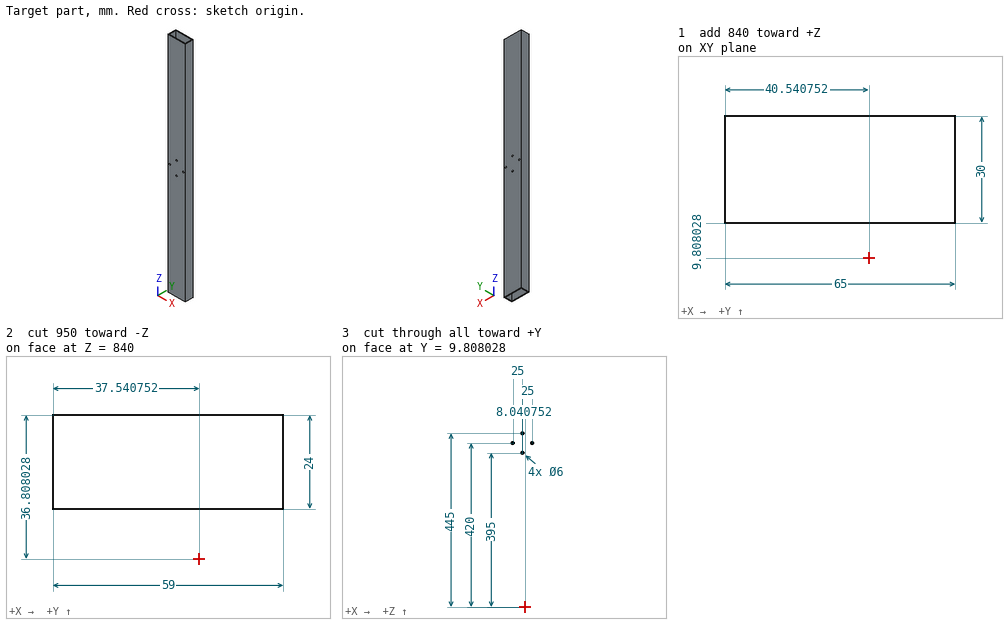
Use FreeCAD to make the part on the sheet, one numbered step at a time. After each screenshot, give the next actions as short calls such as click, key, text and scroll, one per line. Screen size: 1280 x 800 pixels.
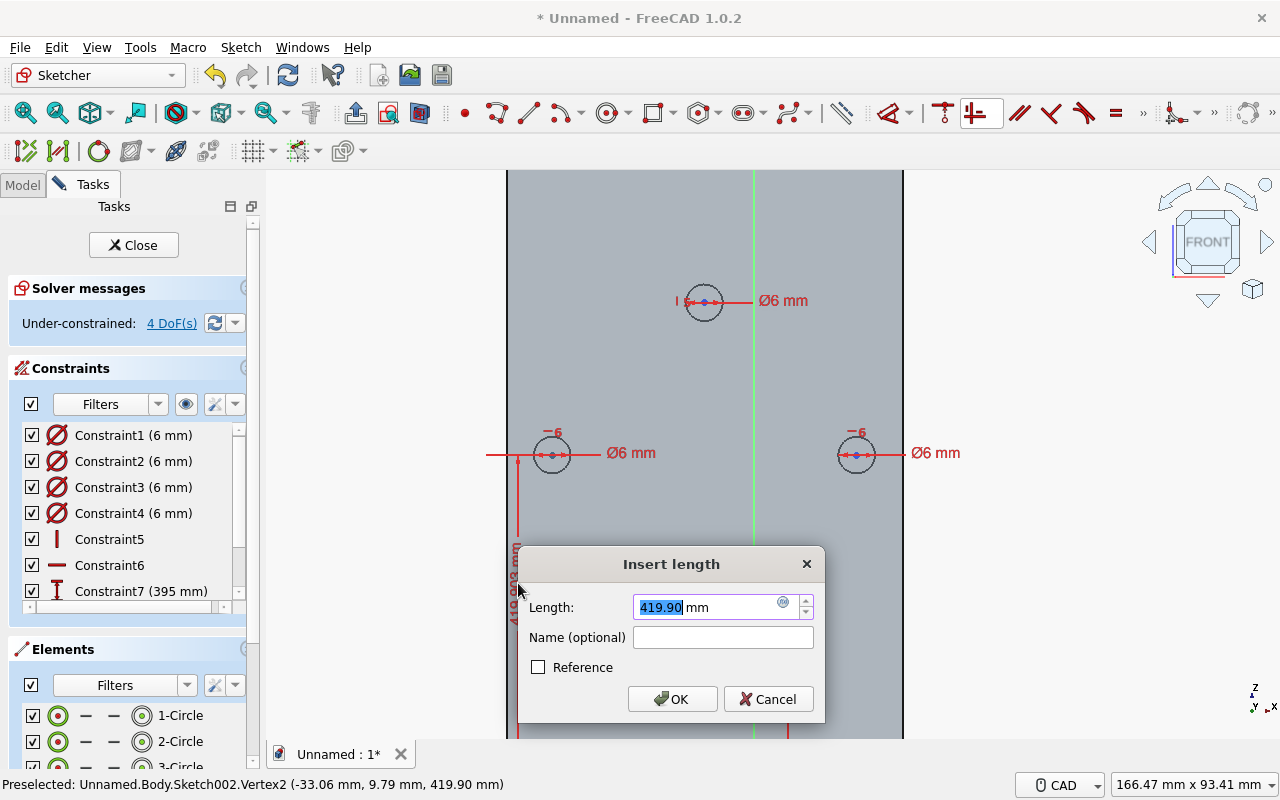
text(420)
key(Return)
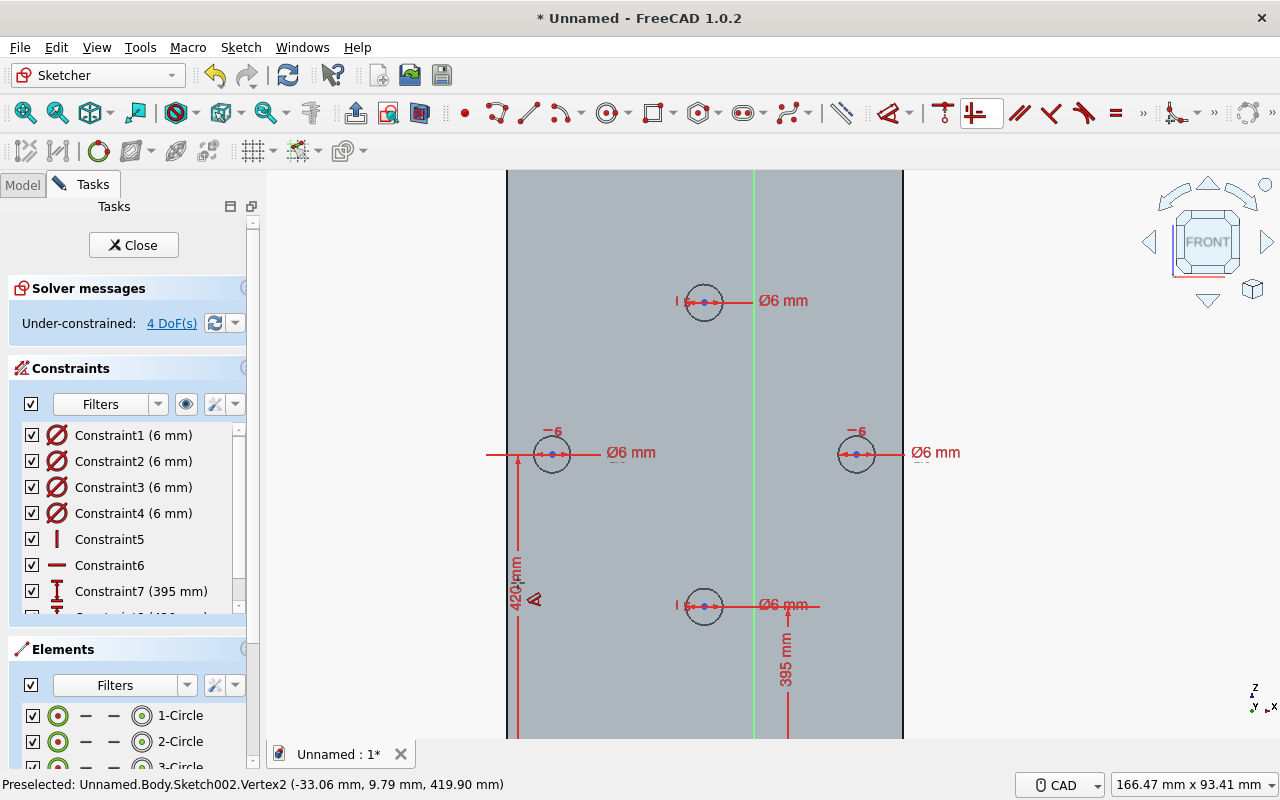
click(704, 303)
click(788, 507)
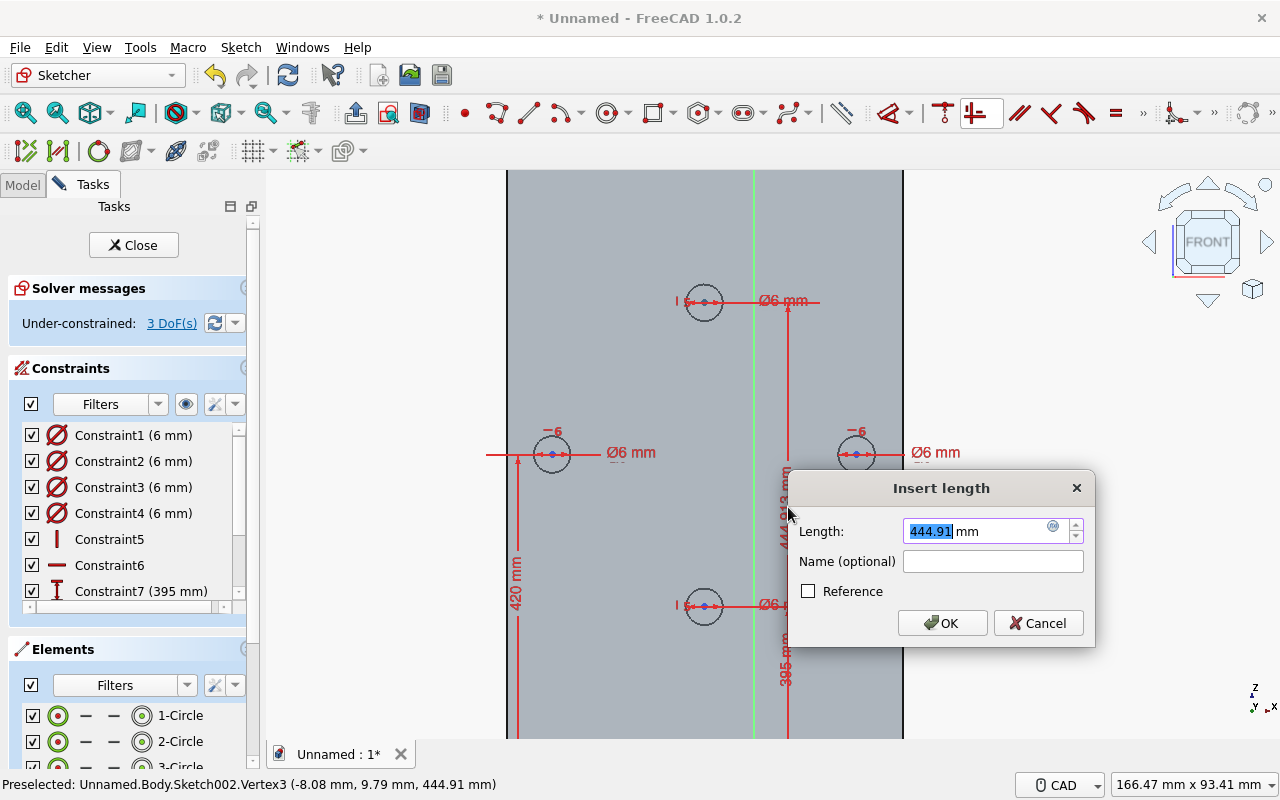
text(445)
key(Return)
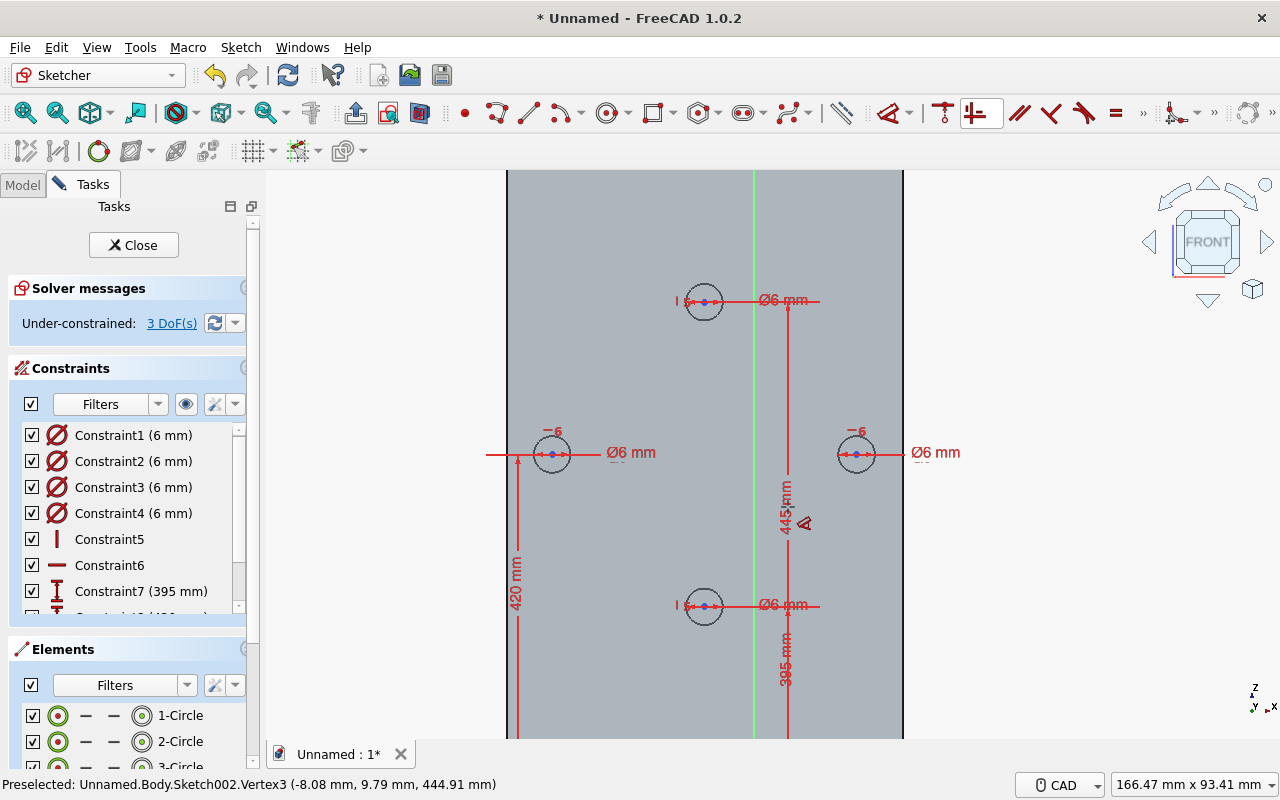
click(704, 607)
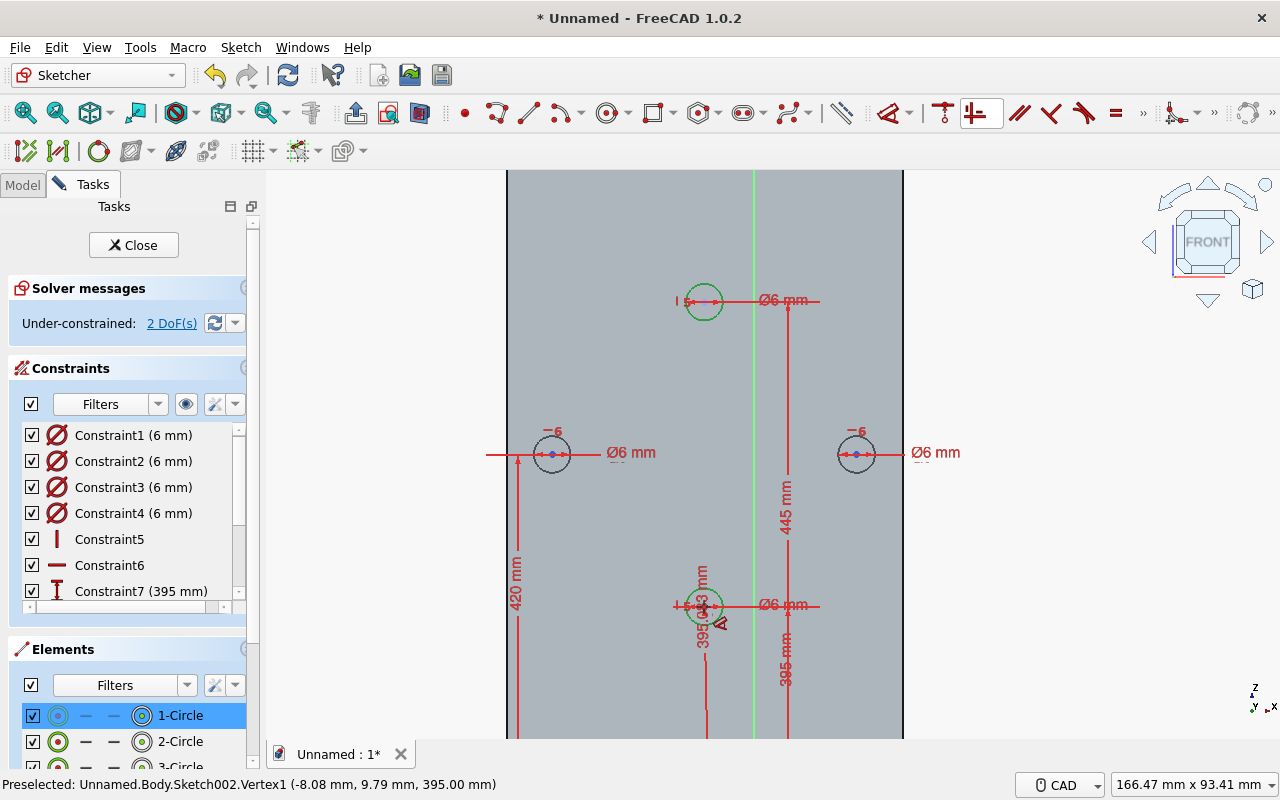
click(552, 454)
click(628, 641)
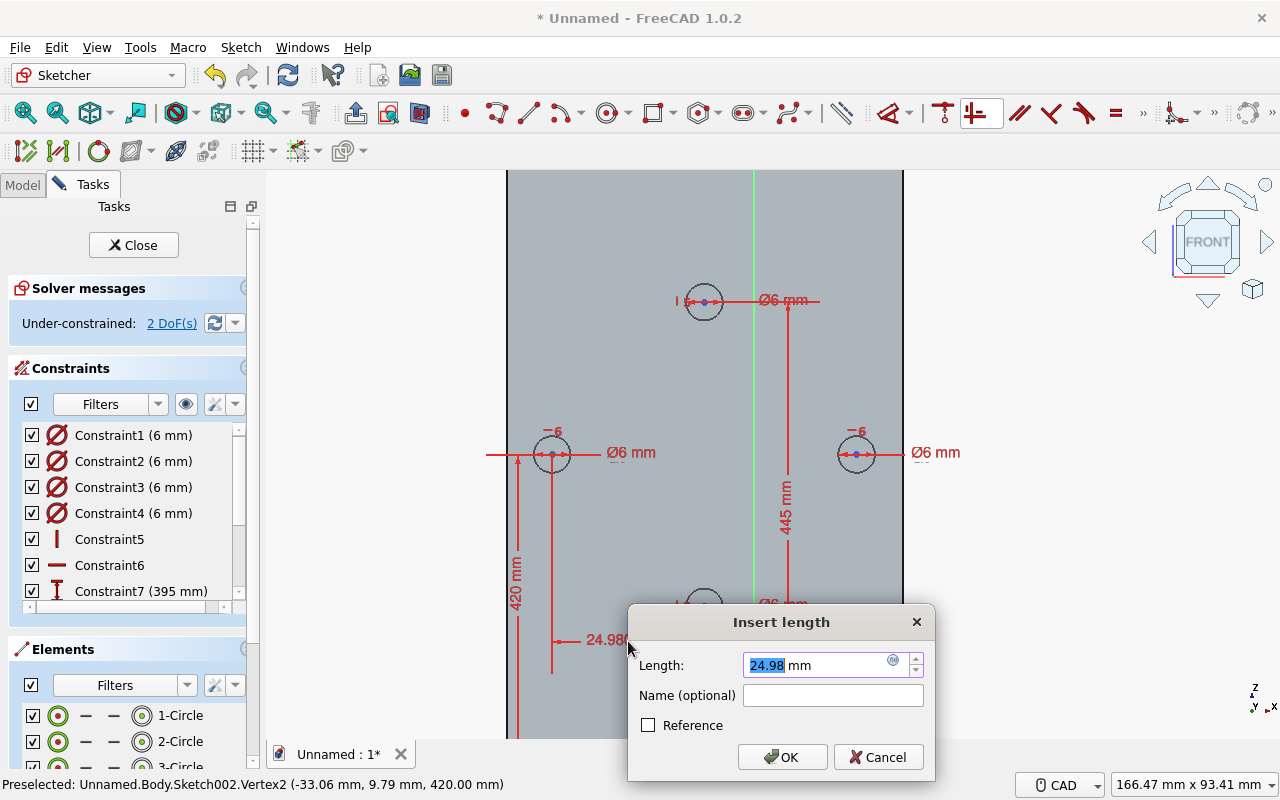
text(25)
key(Return)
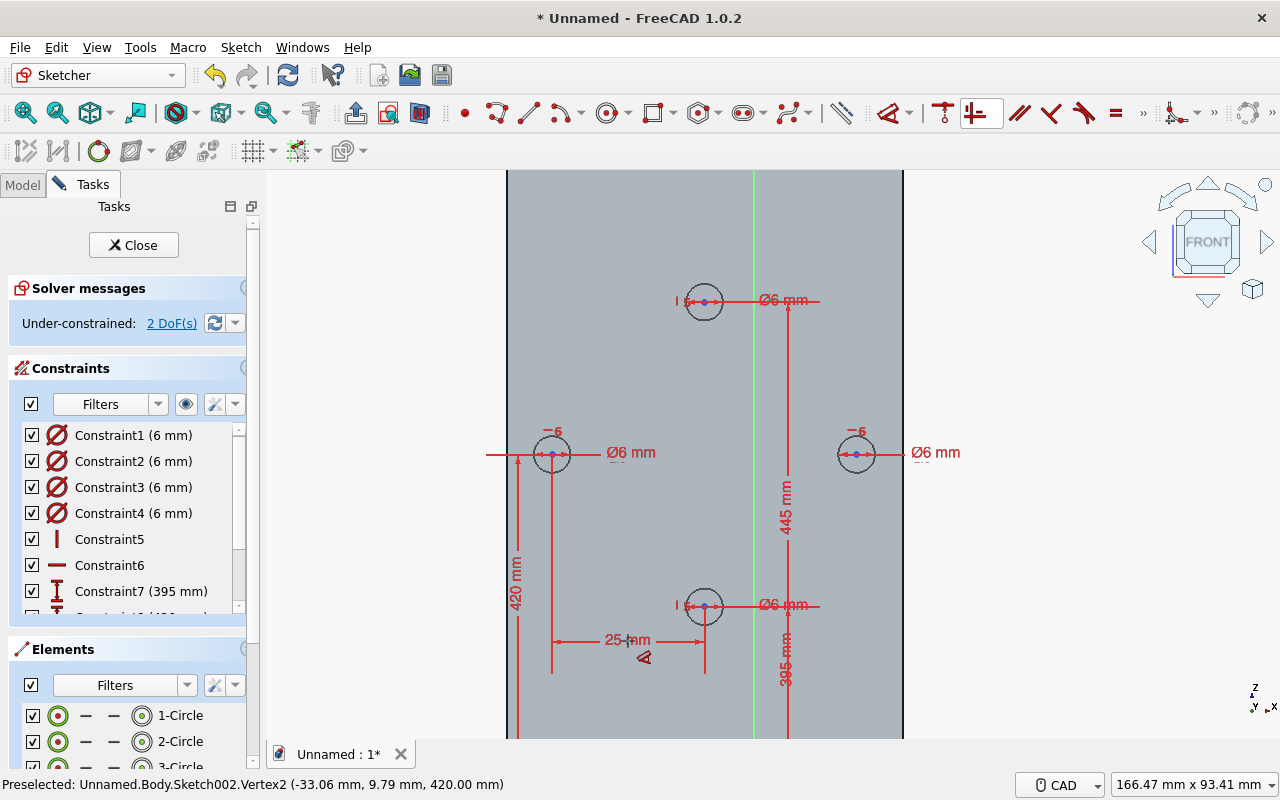
click(705, 607)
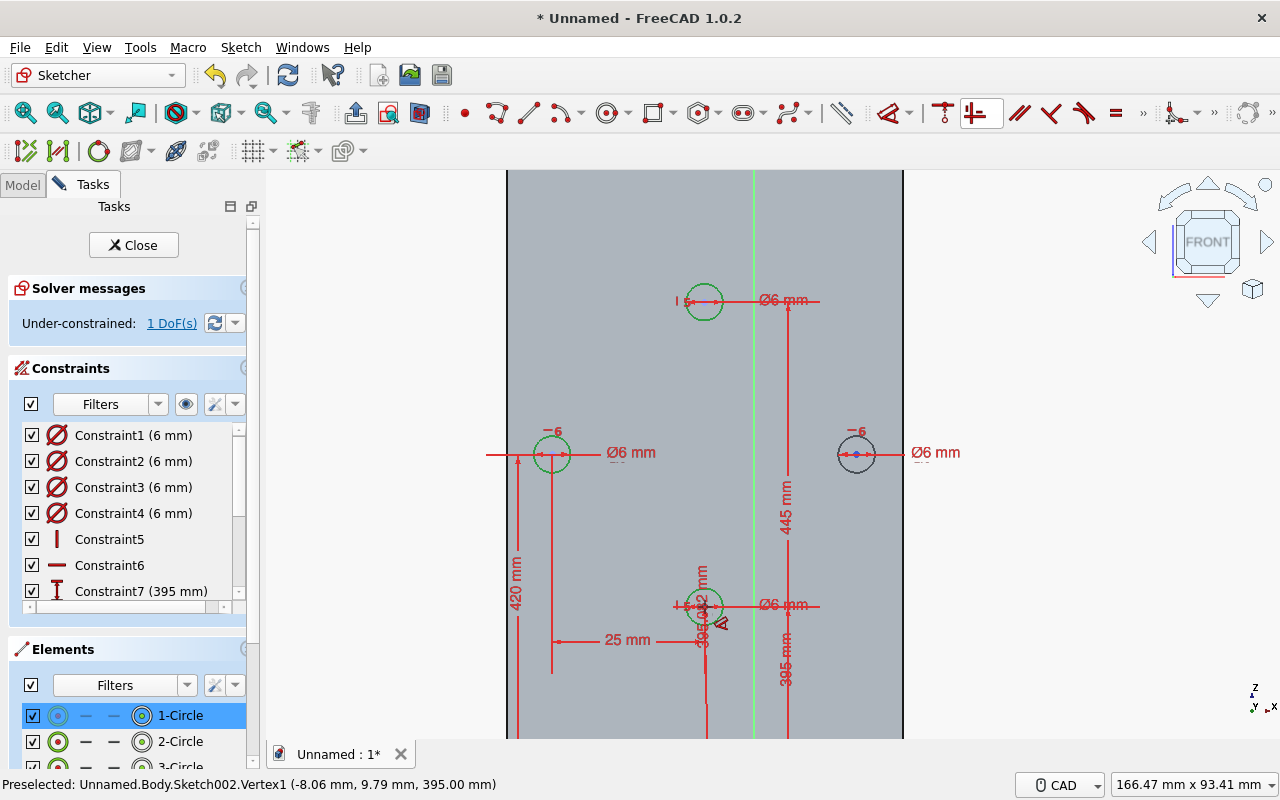
click(857, 454)
click(781, 420)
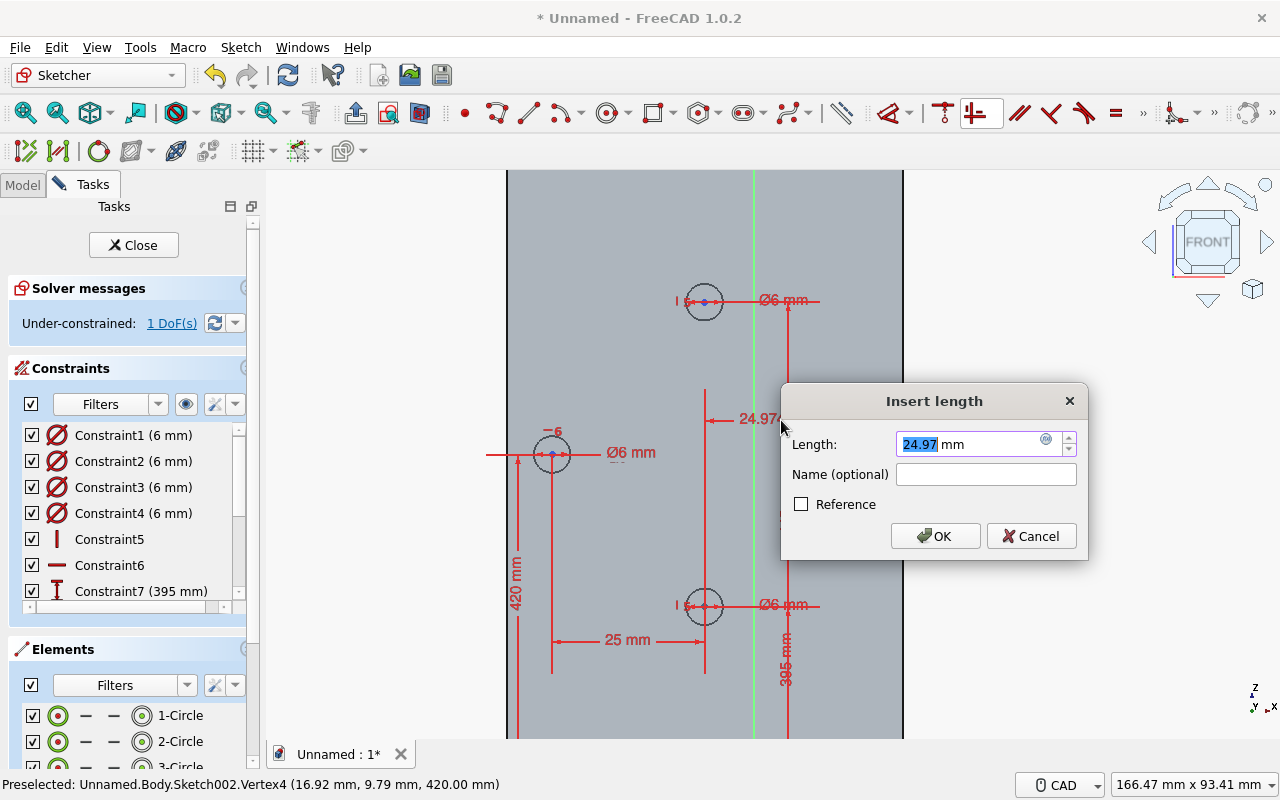
text(25)
key(Return)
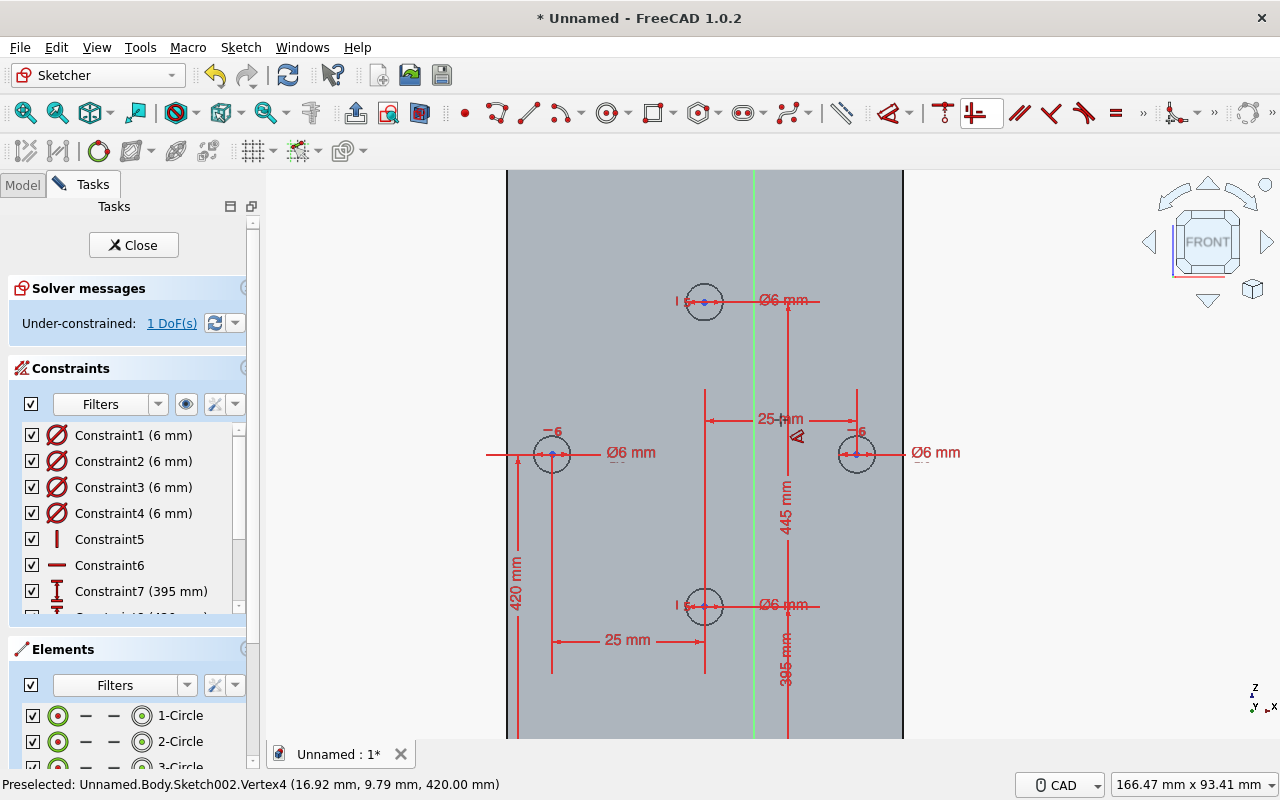
click(705, 607)
click(729, 573)